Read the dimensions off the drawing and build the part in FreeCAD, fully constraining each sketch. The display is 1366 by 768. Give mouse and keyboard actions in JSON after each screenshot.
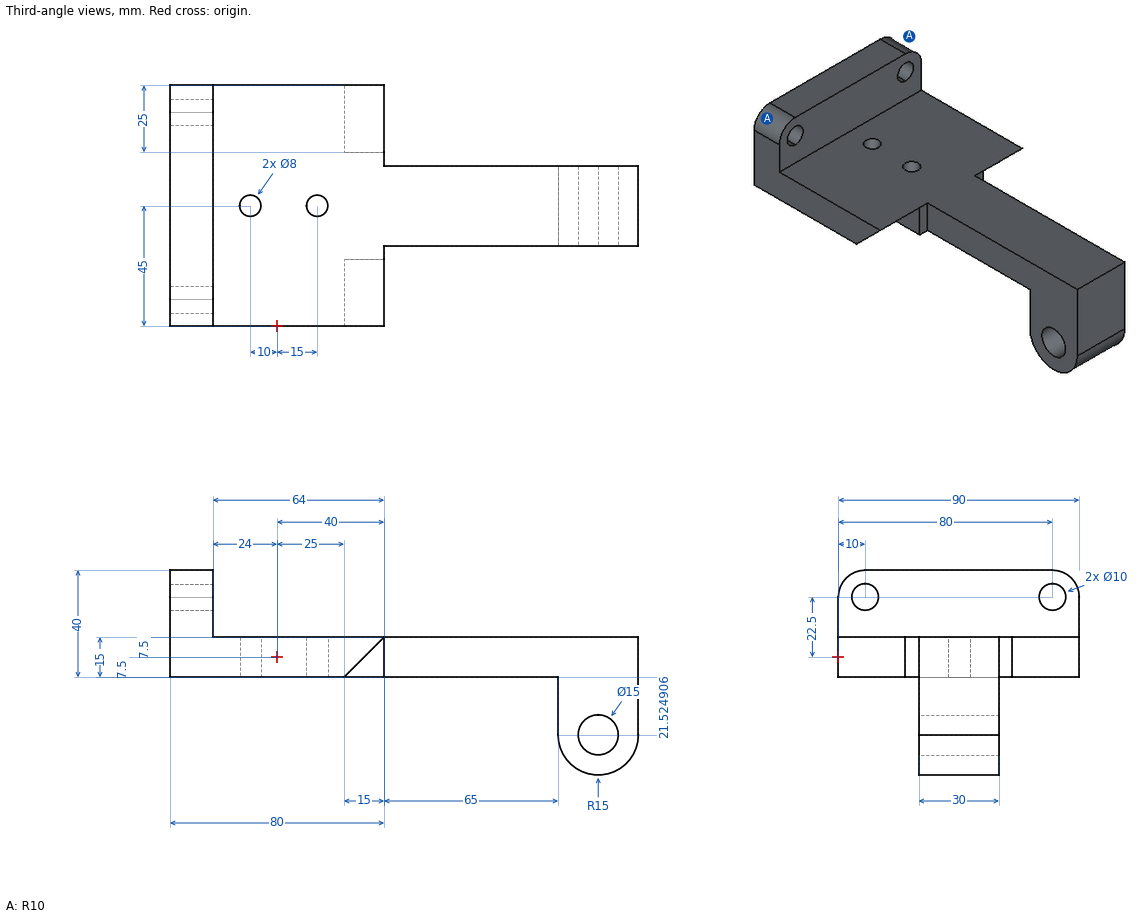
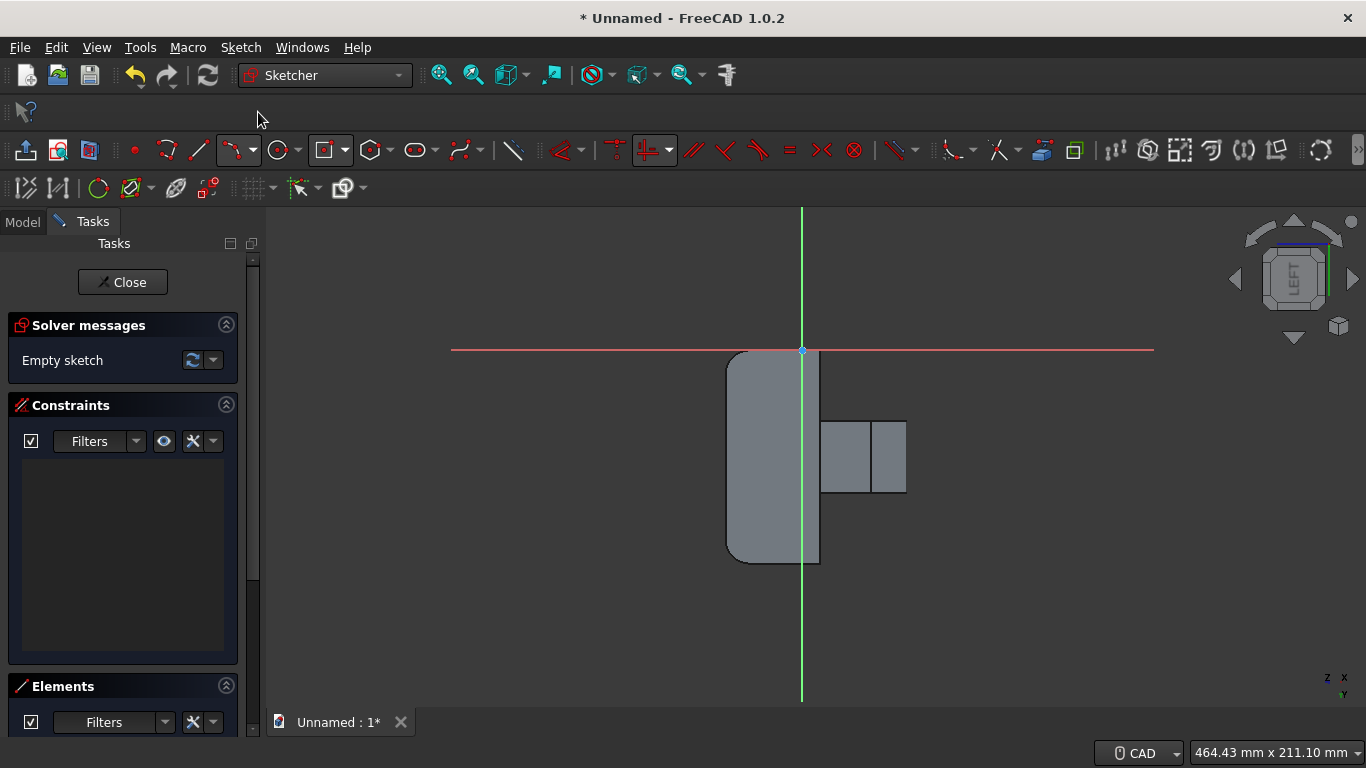
{"action": "scroll", "coordinate": [815, 439], "scroll_direction": "up", "scroll_amount": 2}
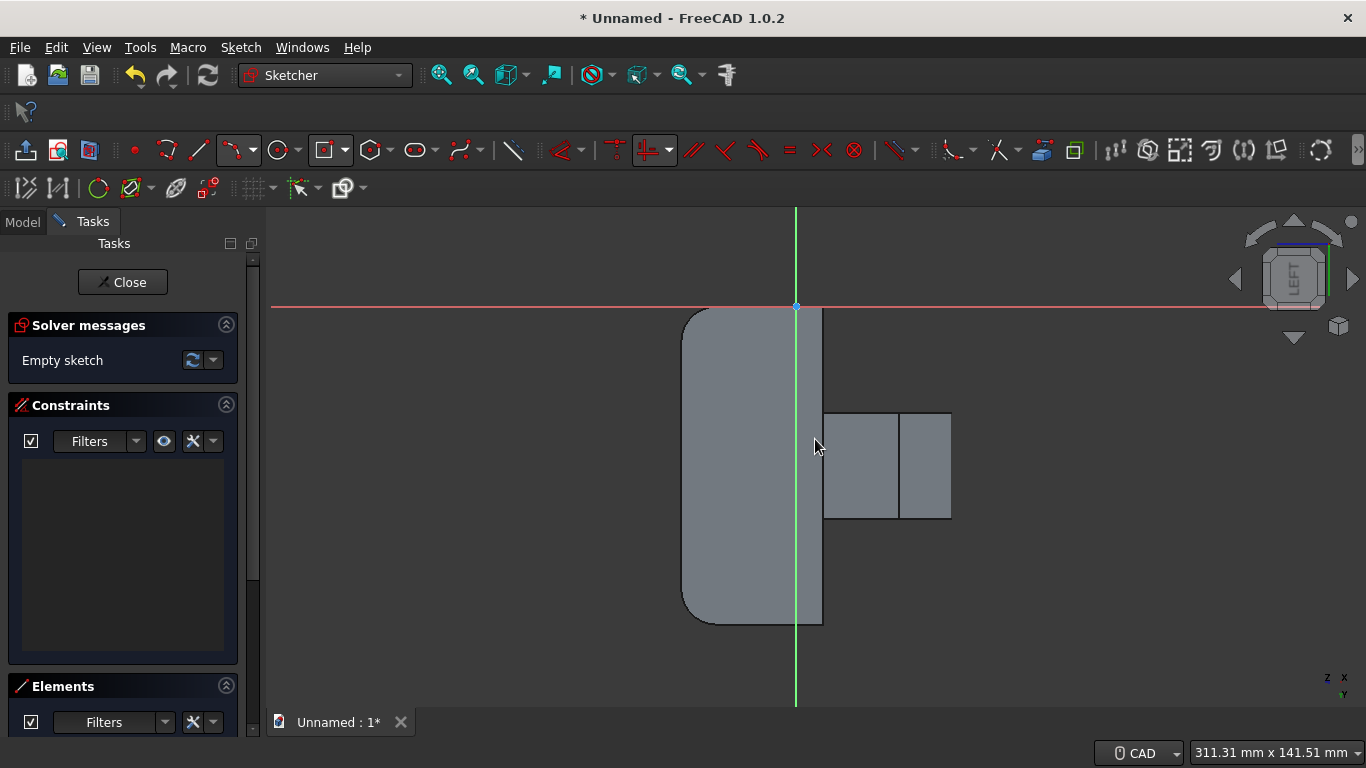
{"action": "left_click", "coordinate": [278, 150]}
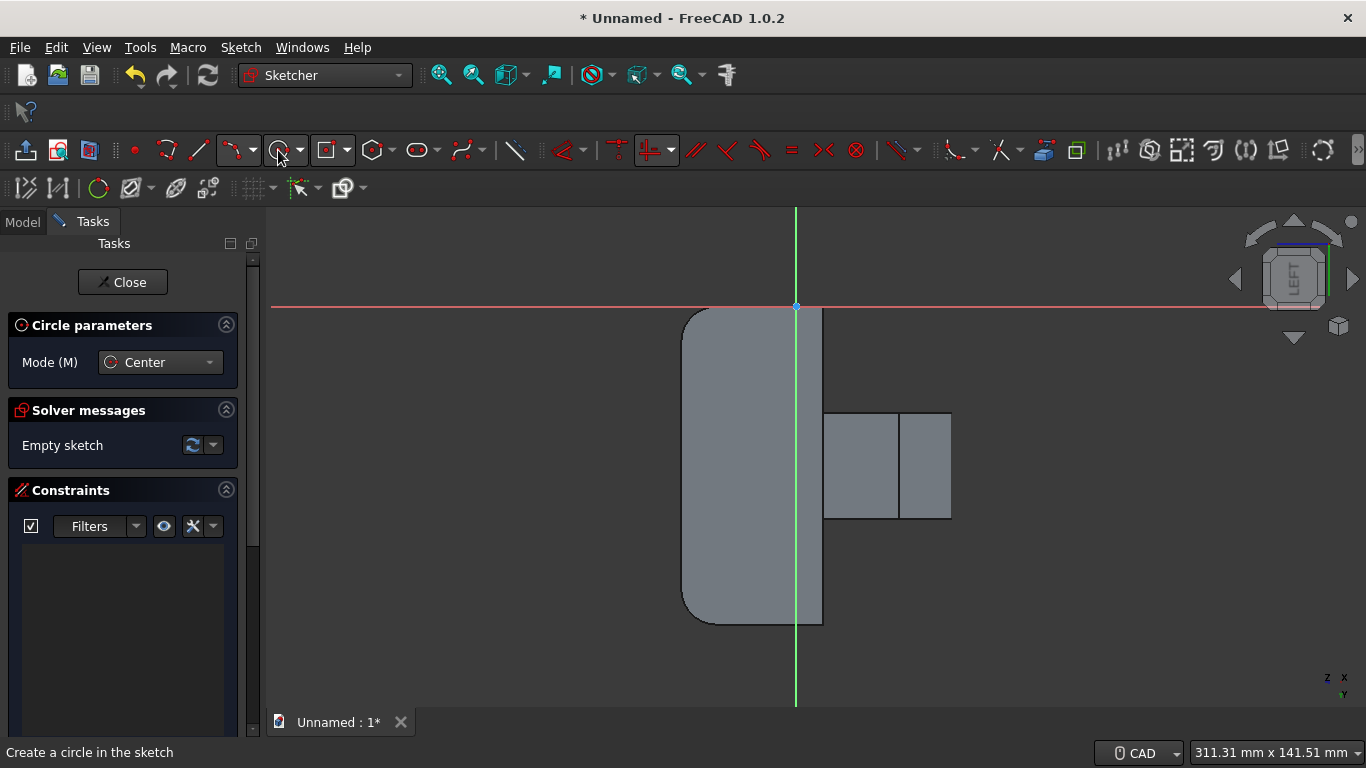
{"action": "scroll", "coordinate": [717, 589], "scroll_direction": "up", "scroll_amount": 2}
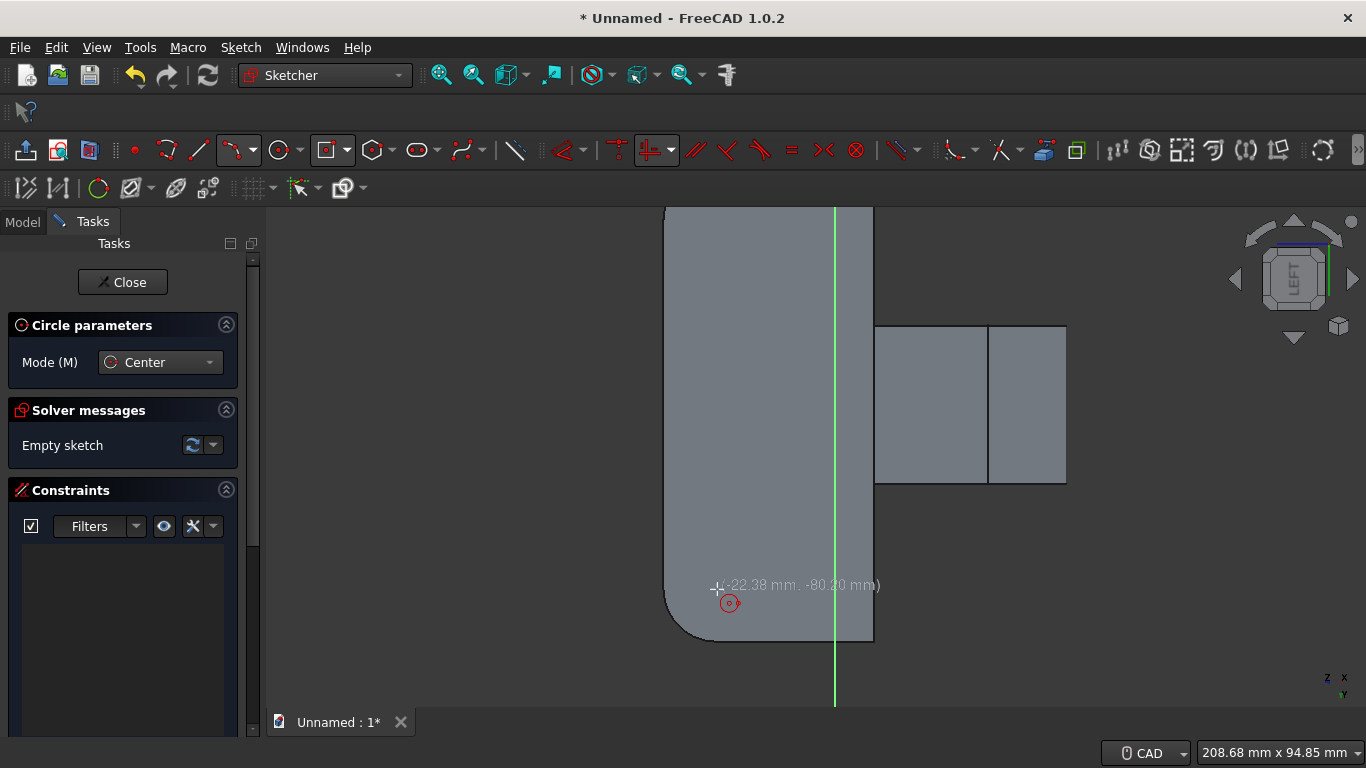
{"action": "left_click", "coordinate": [716, 589]}
{"action": "left_click", "coordinate": [735, 570]}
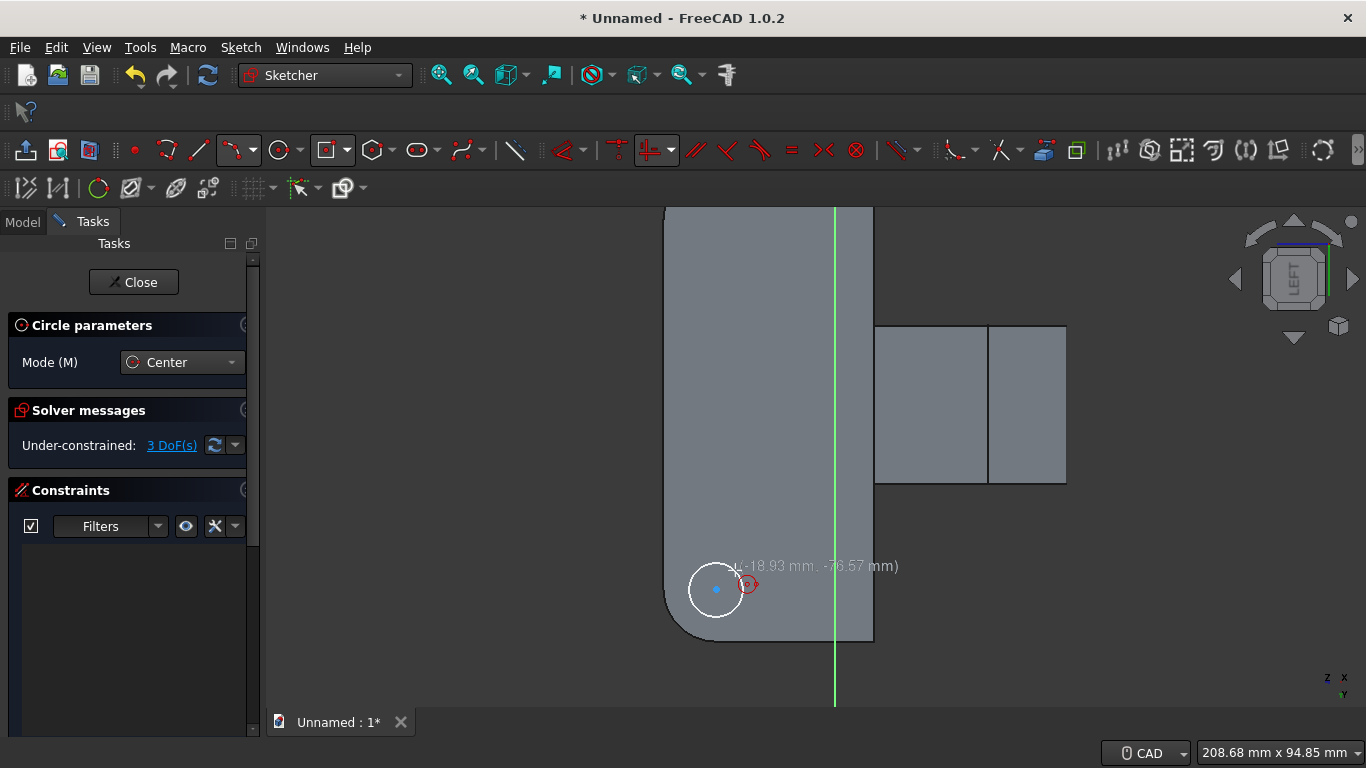
{"action": "scroll", "coordinate": [717, 590], "scroll_direction": "down", "scroll_amount": 2}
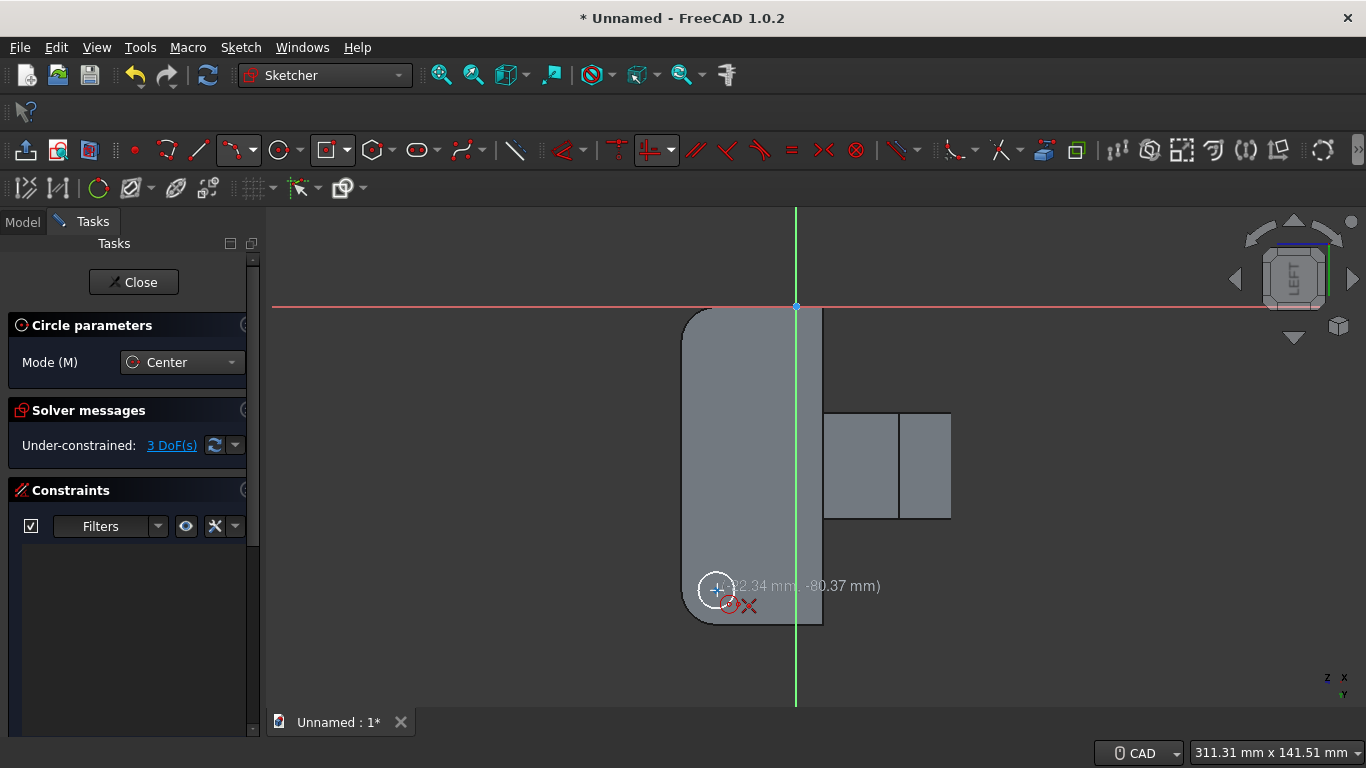
{"action": "scroll", "coordinate": [717, 342], "scroll_direction": "up", "scroll_amount": 2}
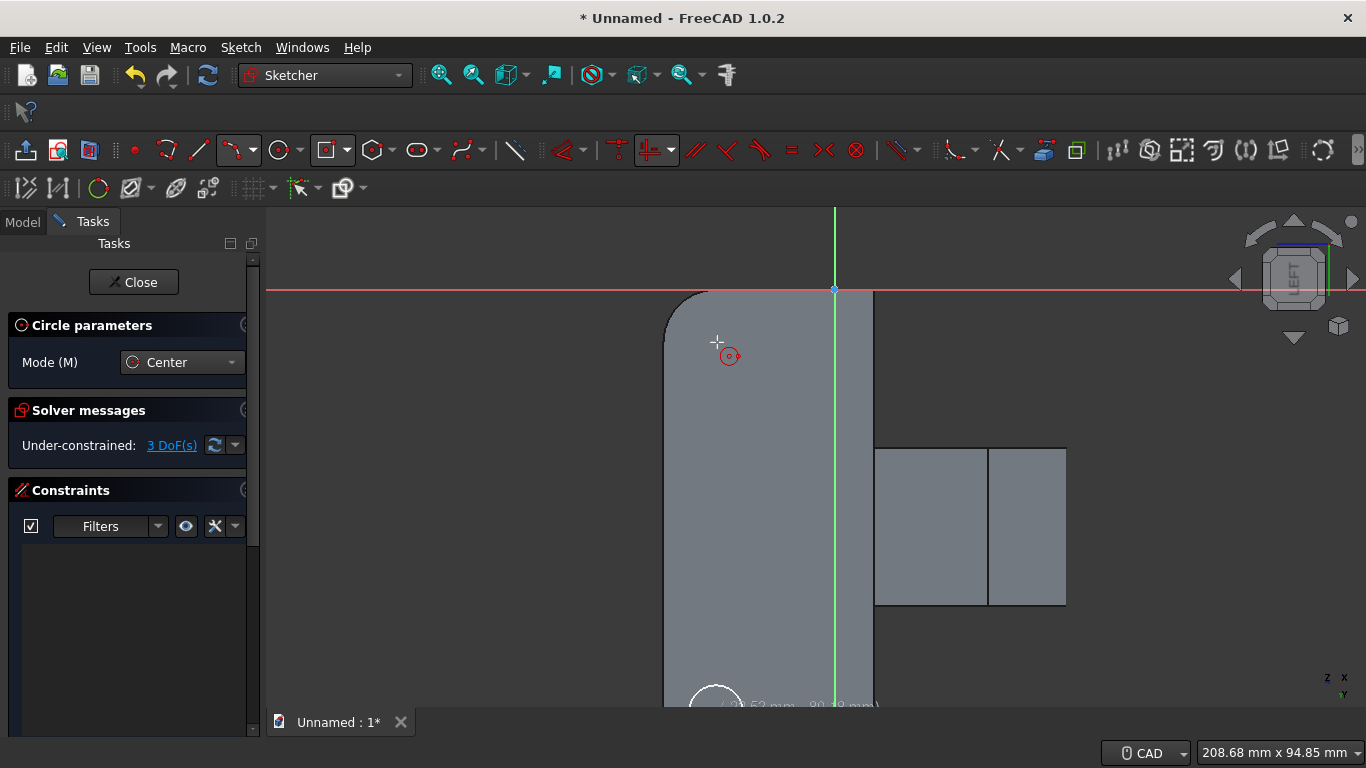
{"action": "left_click", "coordinate": [716, 342]}
{"action": "left_click", "coordinate": [735, 324]}
{"action": "key", "text": "Escape"}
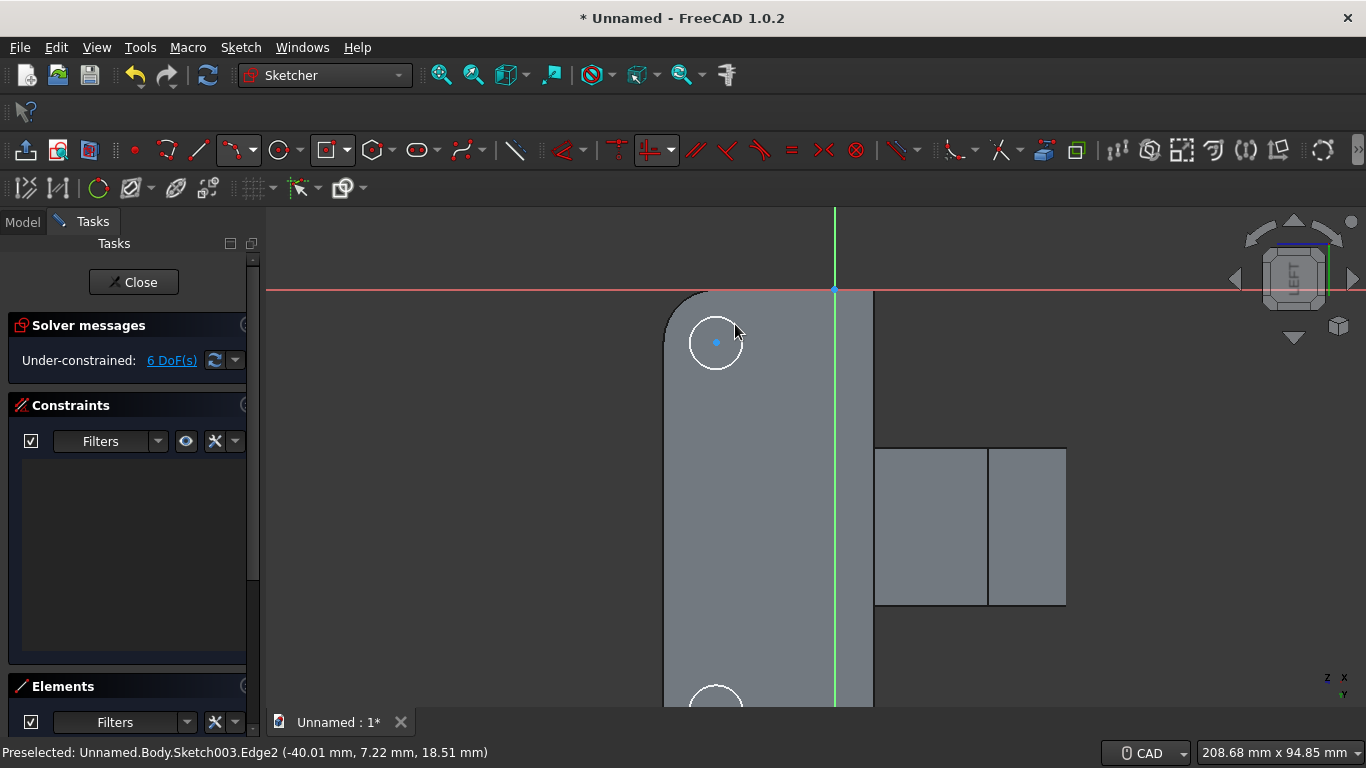
{"action": "scroll", "coordinate": [717, 342], "scroll_direction": "down", "scroll_amount": 2}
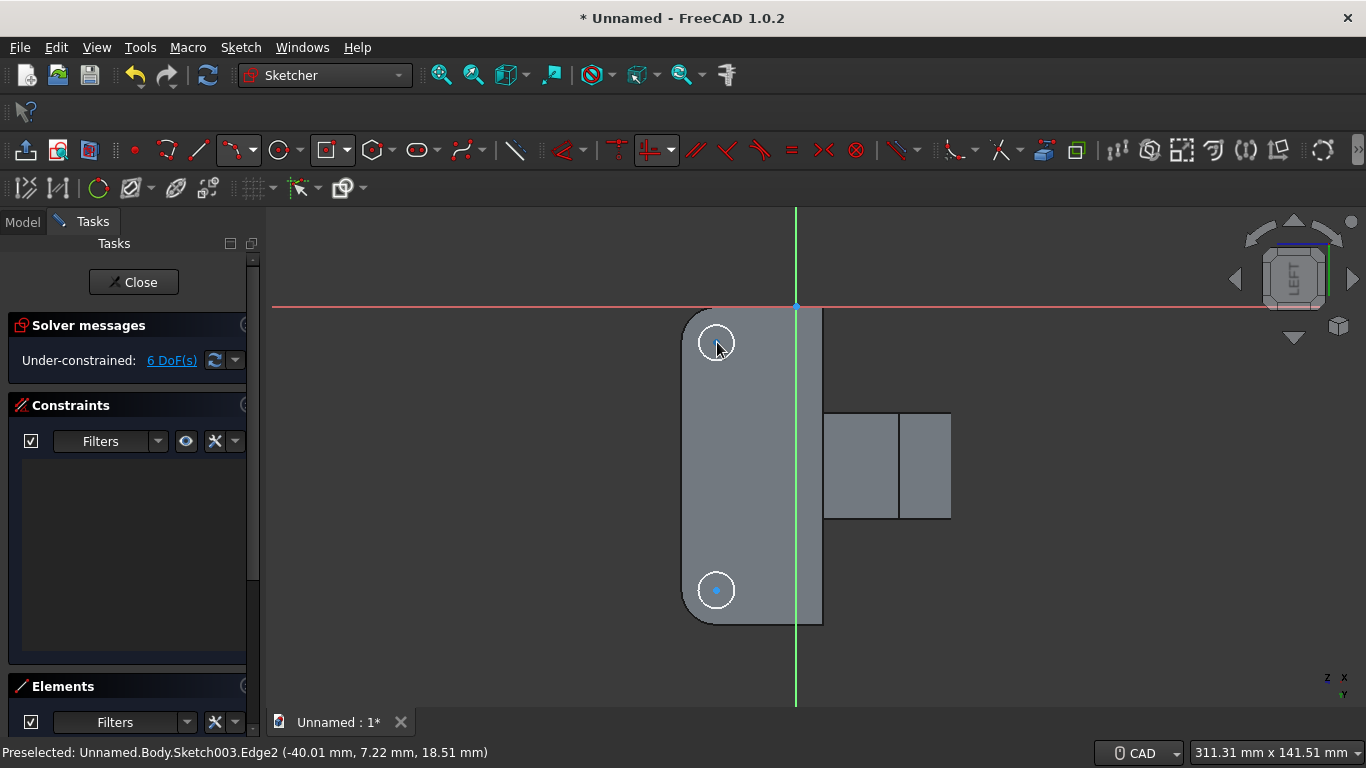
{"action": "left_click", "coordinate": [729, 577]}